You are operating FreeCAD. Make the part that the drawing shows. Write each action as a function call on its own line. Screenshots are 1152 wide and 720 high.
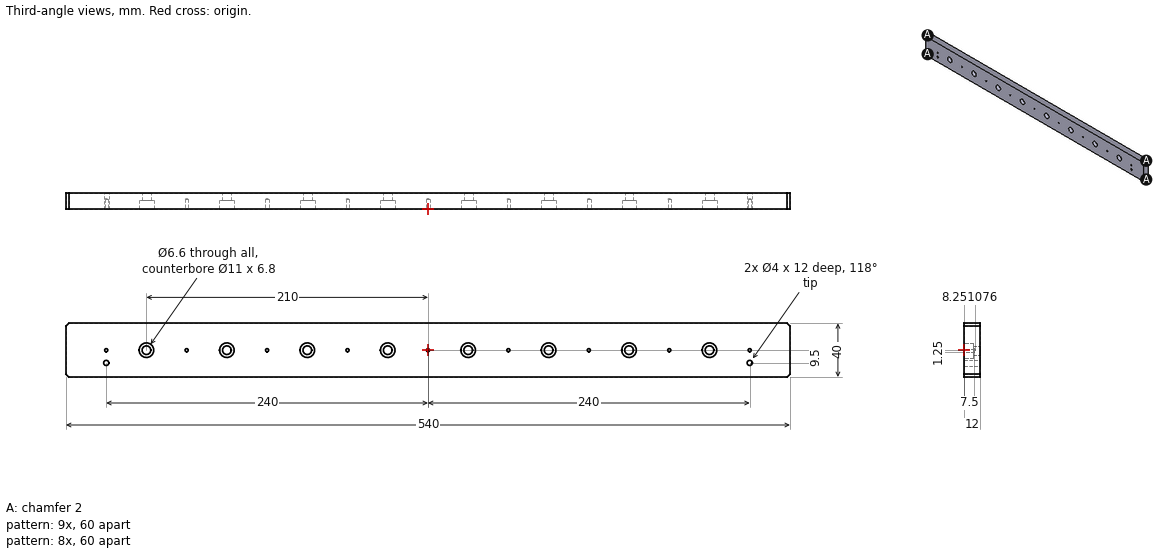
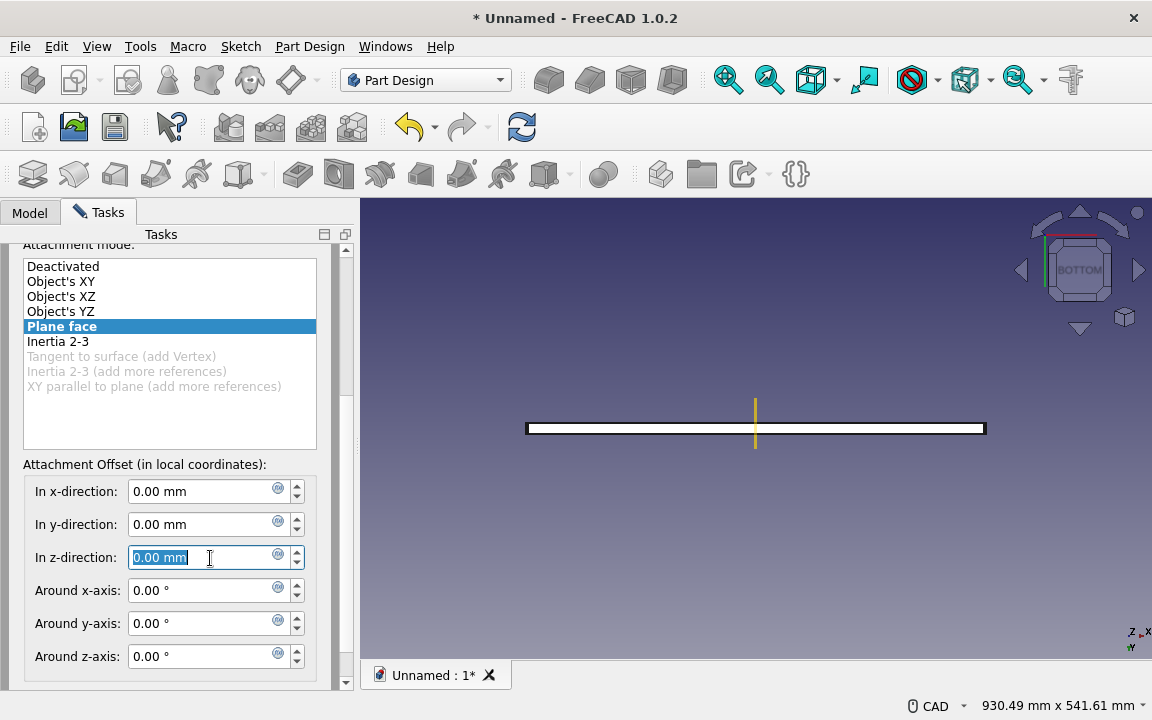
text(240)
key(Tab)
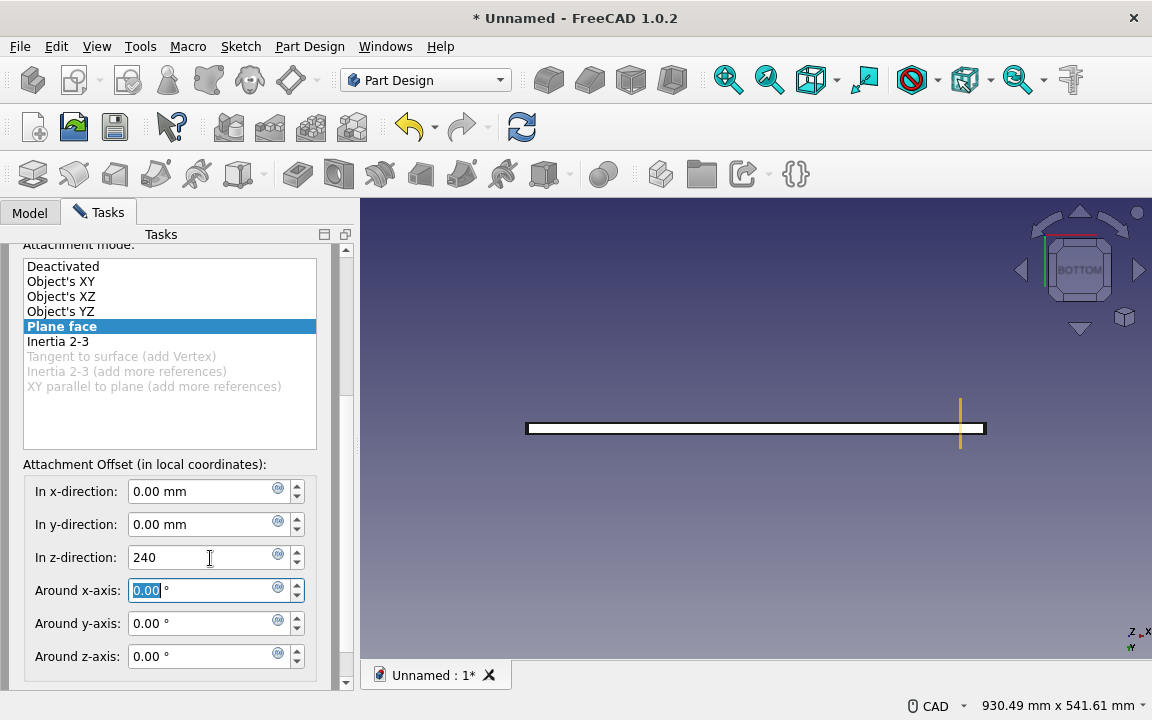
scroll(346, 467, up, 5)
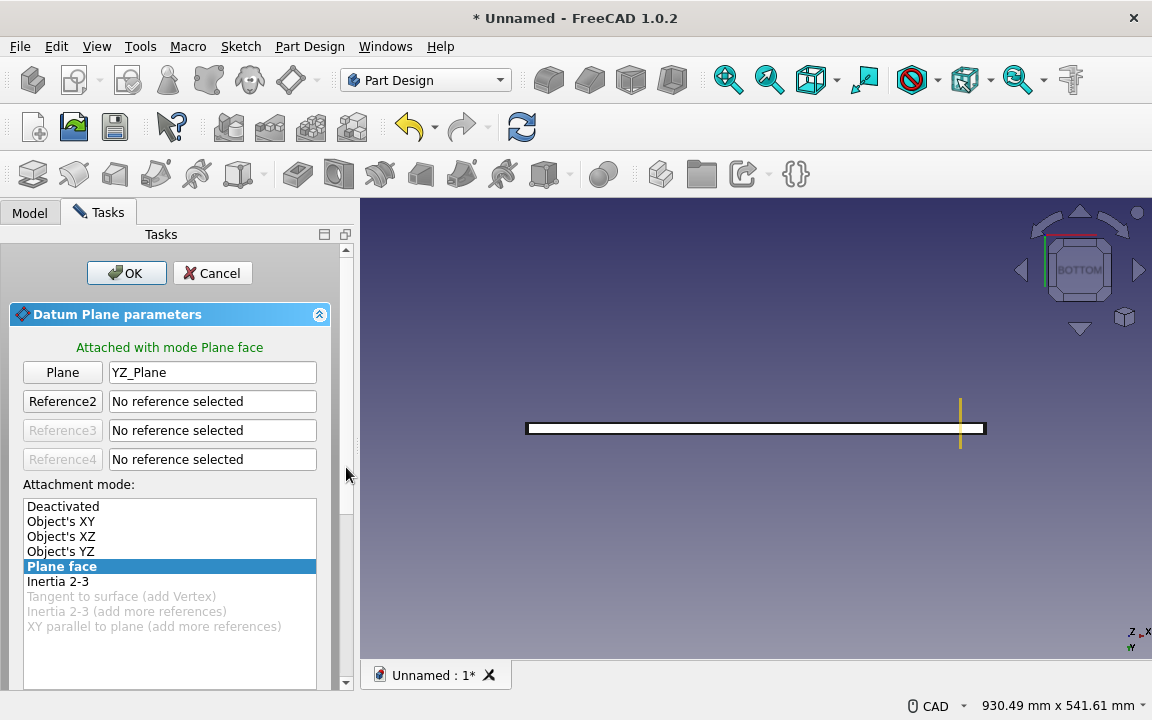
click(127, 273)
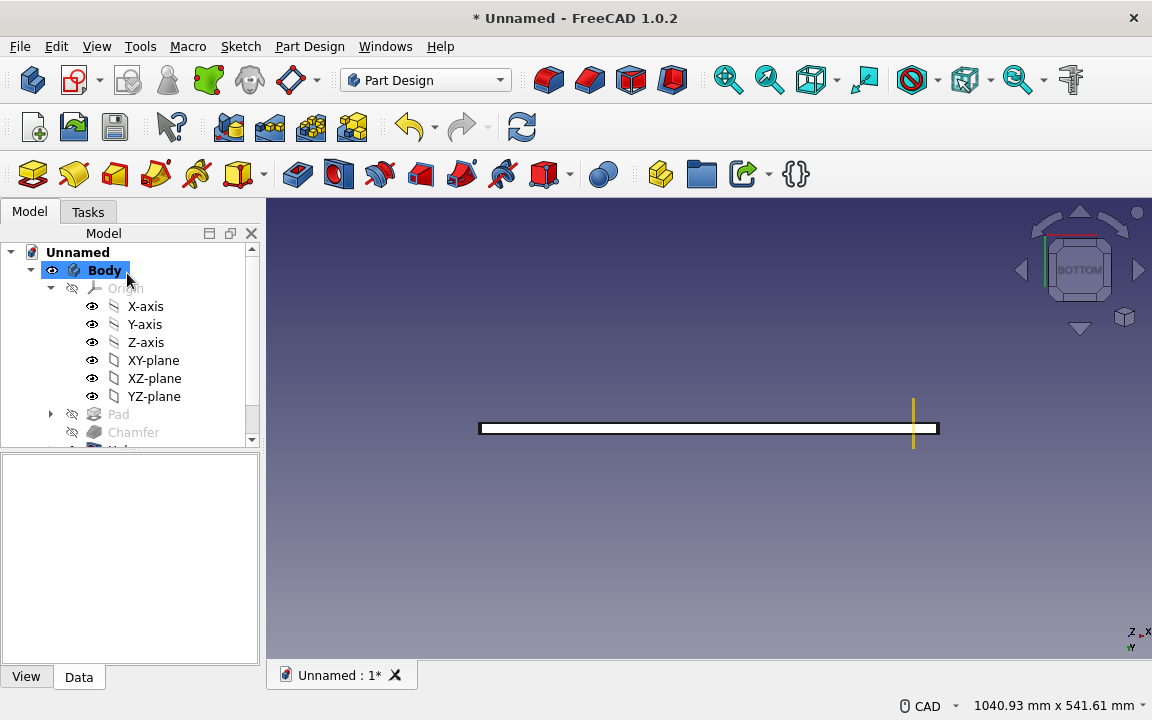
scroll(101, 338, down, 3)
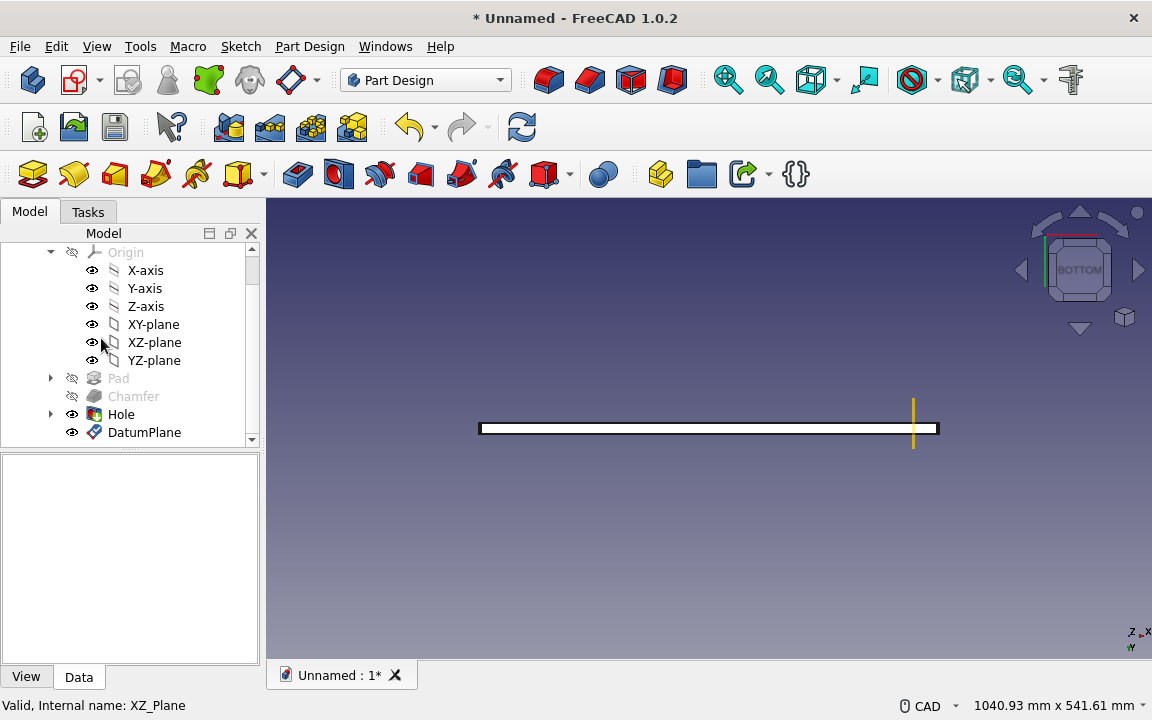
click(117, 432)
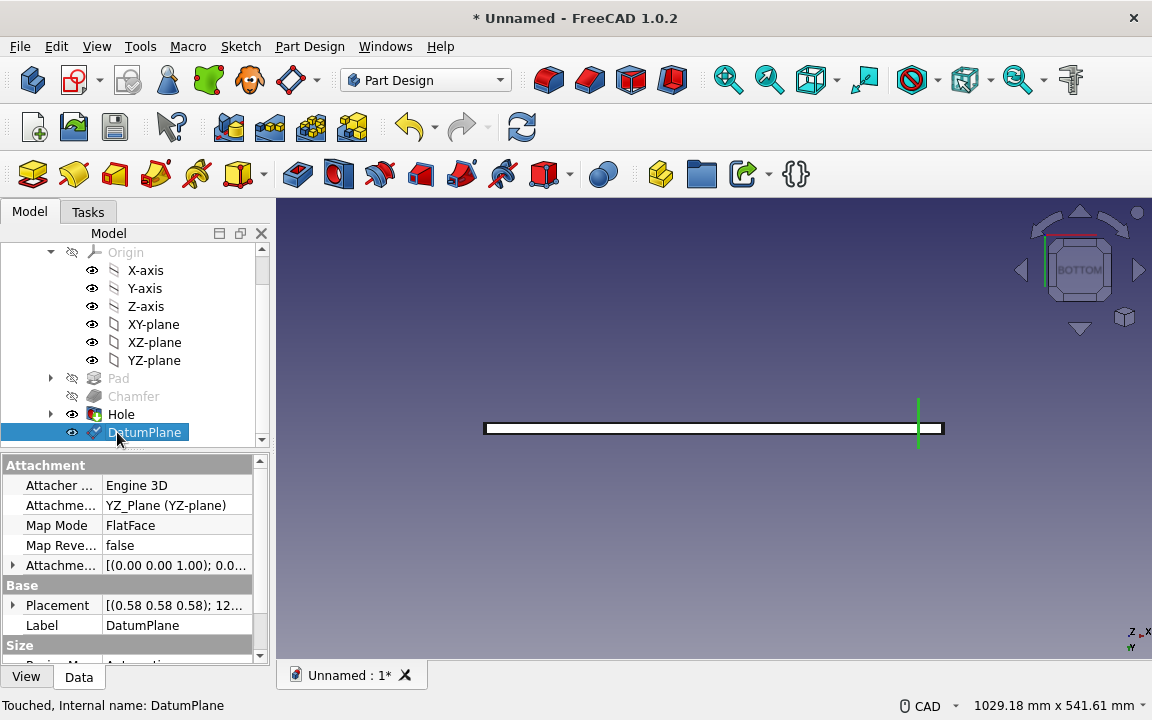
click(74, 80)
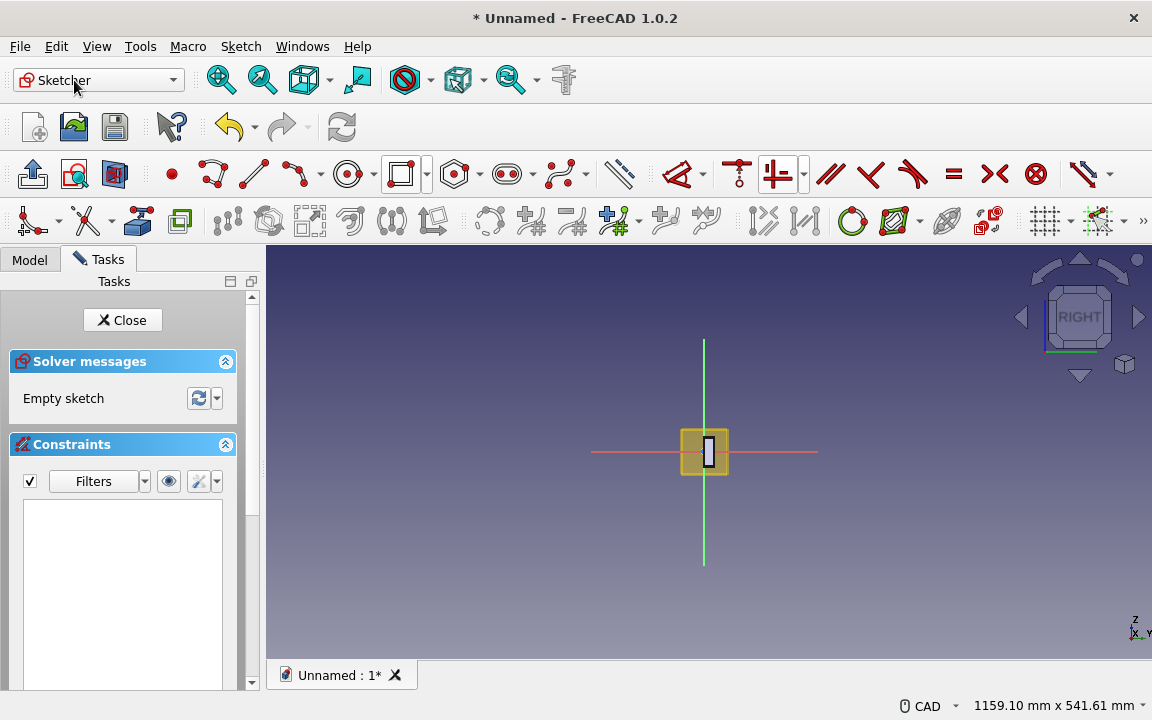
click(115, 174)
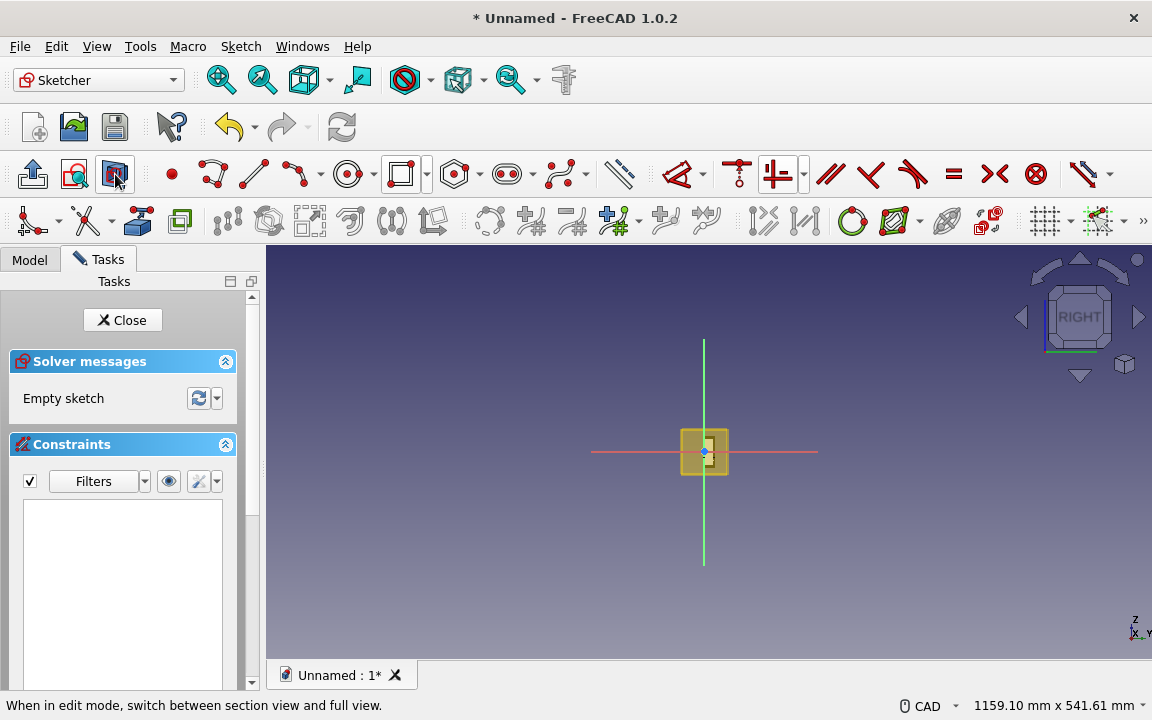
scroll(711, 453, up, 15)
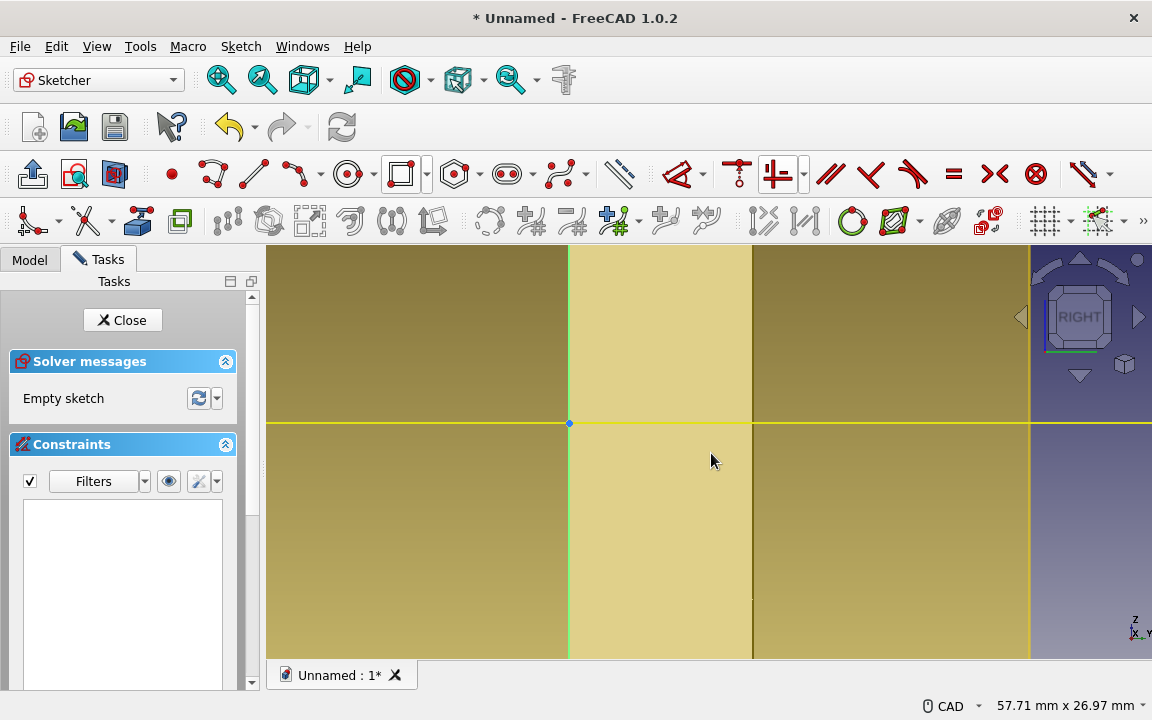
scroll(630, 427, up, 7)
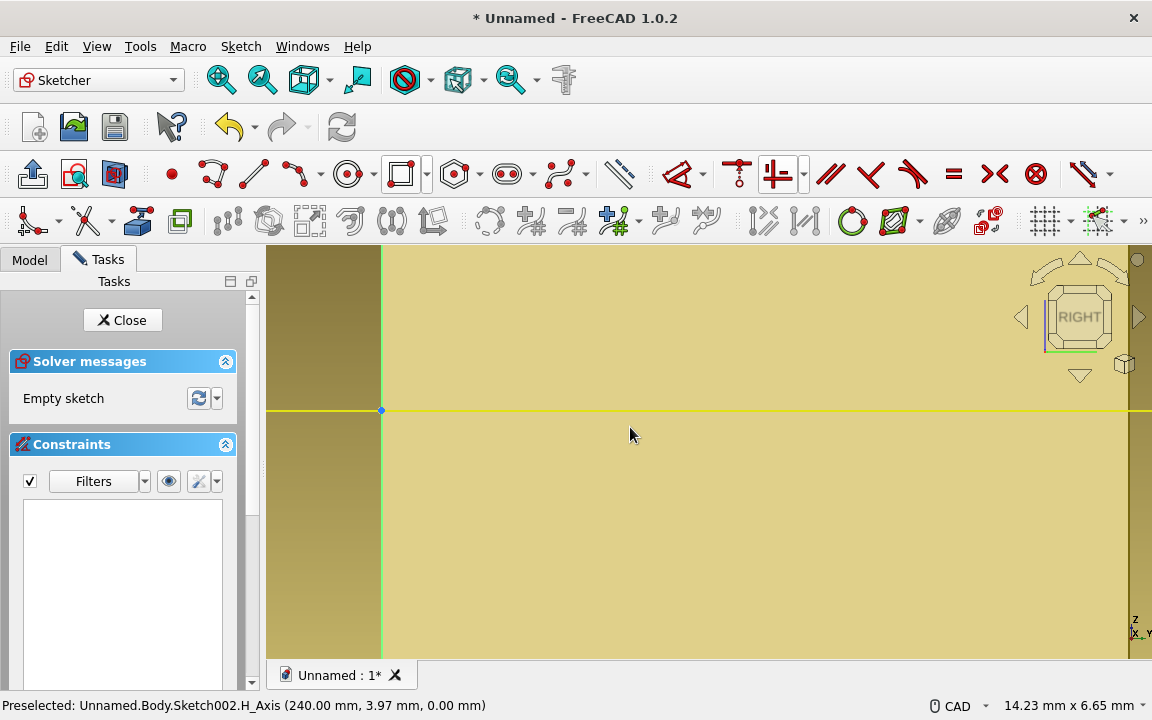
click(213, 174)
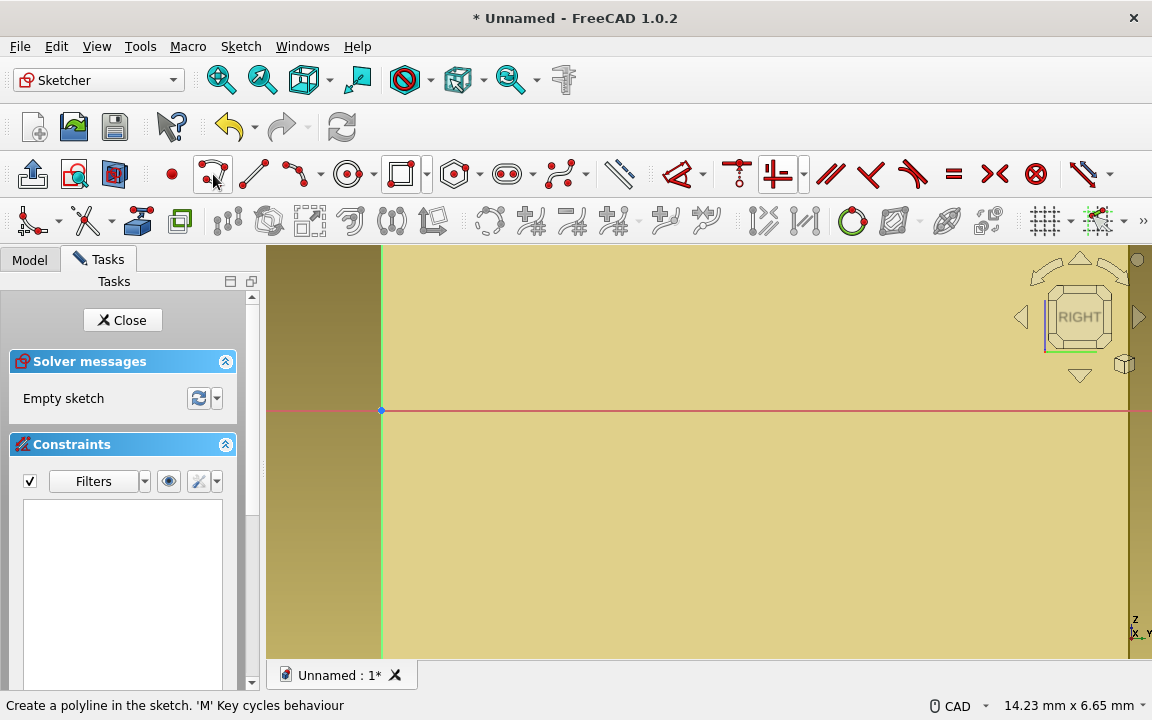
click(382, 411)
click(391, 488)
click(849, 488)
click(896, 420)
click(382, 411)
key(Escape)
key(Escape)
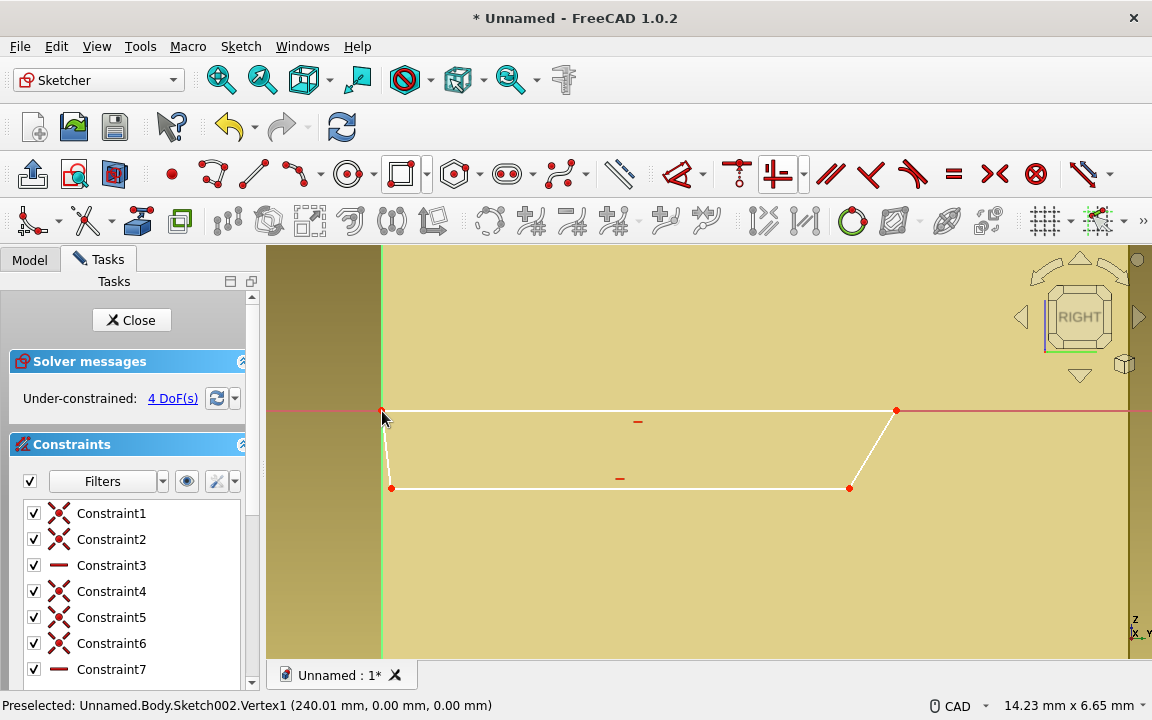
click(385, 434)